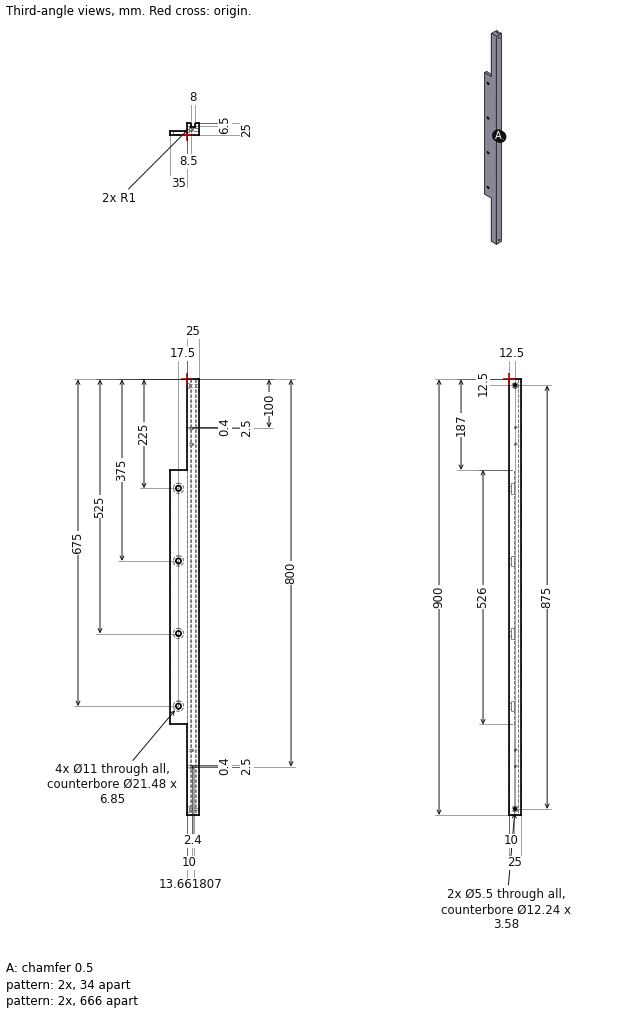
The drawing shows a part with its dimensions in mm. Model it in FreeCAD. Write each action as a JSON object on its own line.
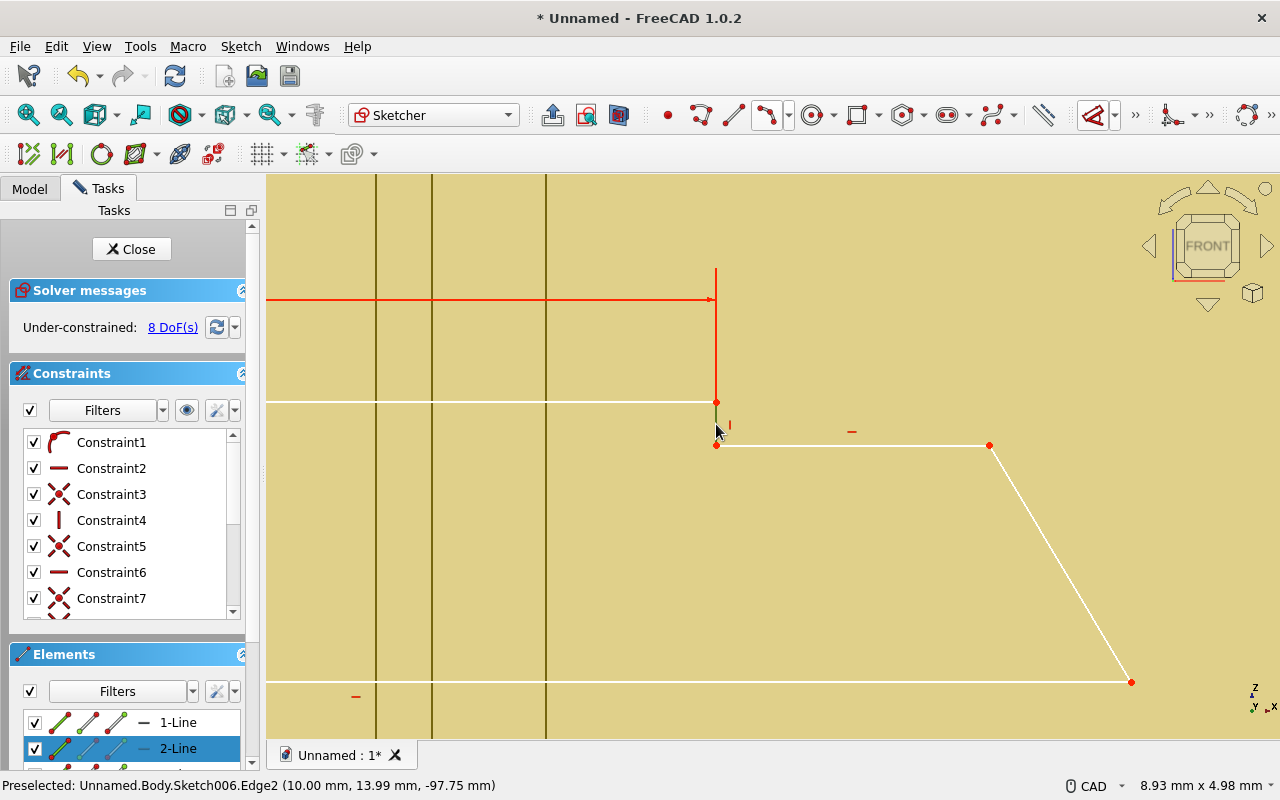
{"action": "left_click", "coordinate": [1114, 116]}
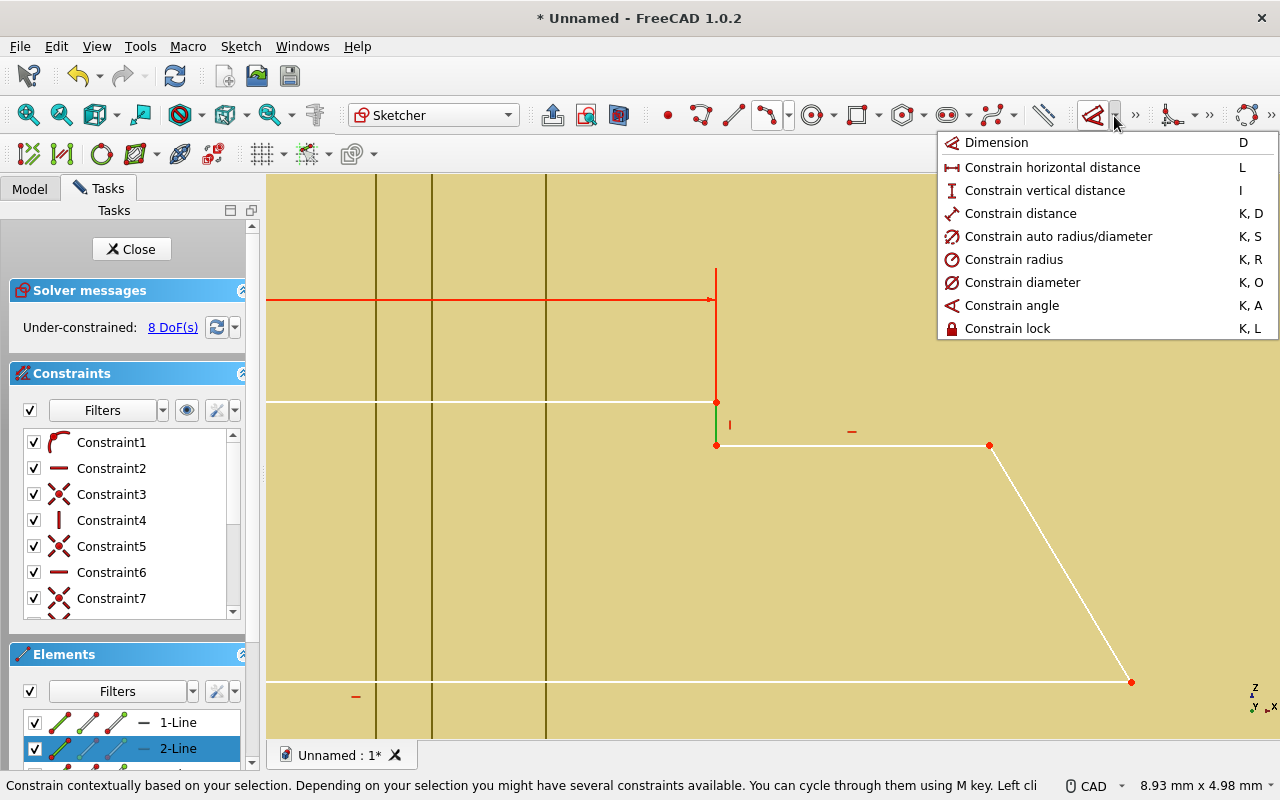
{"action": "left_click", "coordinate": [1108, 190]}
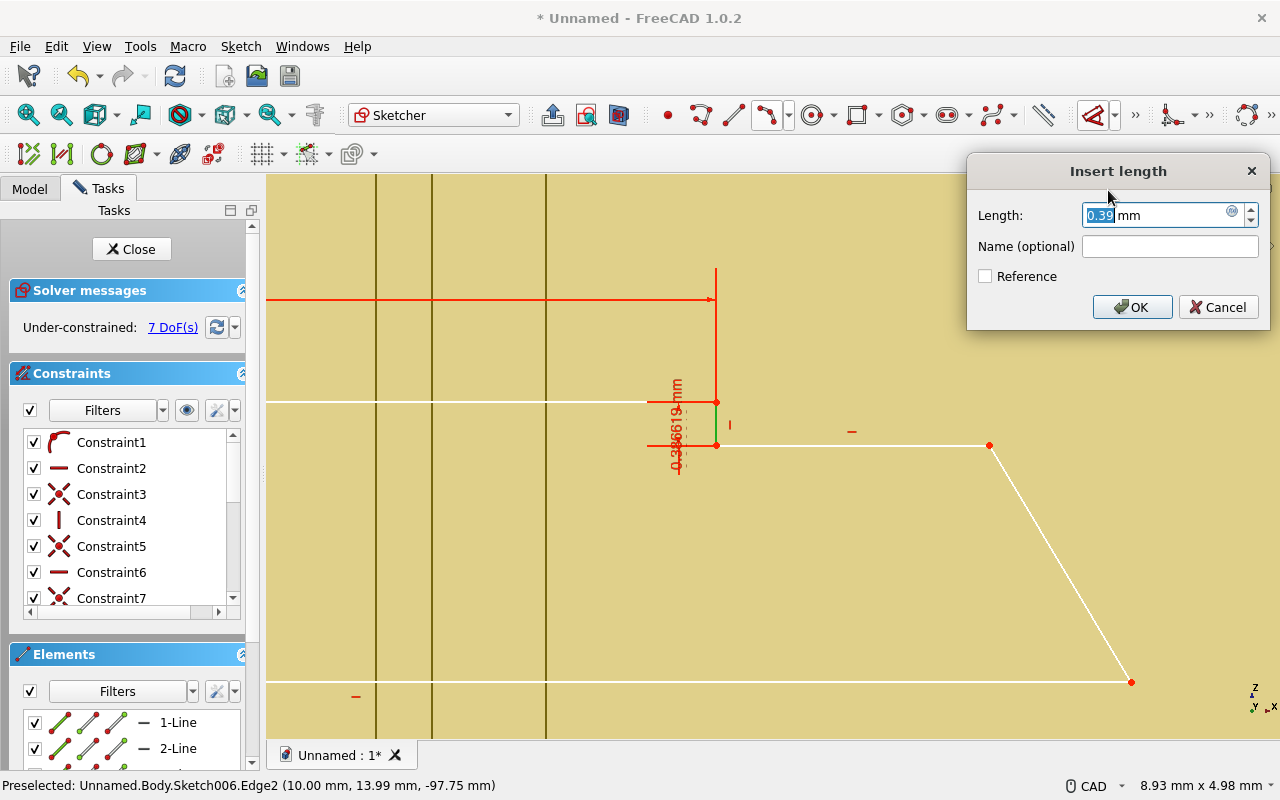
{"action": "type", "text": "0.4"}
{"action": "key", "text": "Return"}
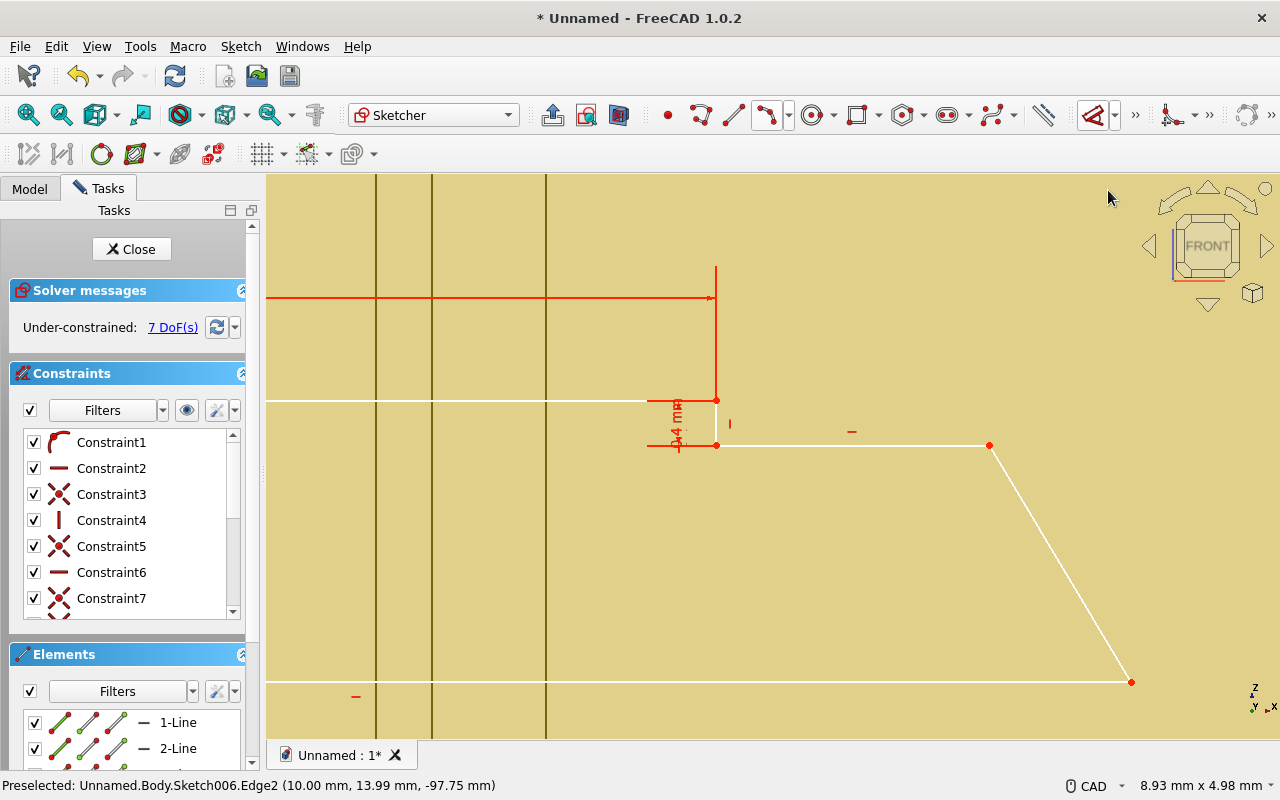
{"action": "scroll", "coordinate": [717, 430], "scroll_direction": "down", "scroll_amount": 7}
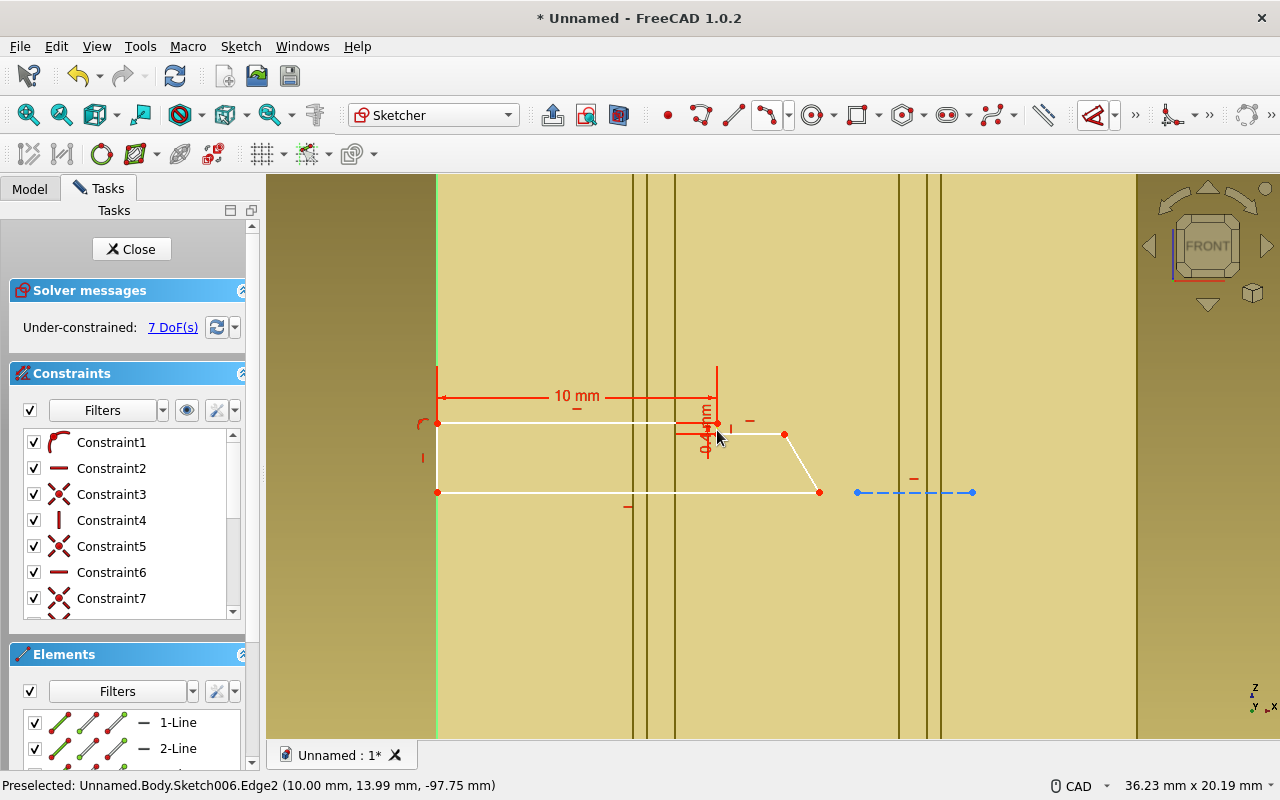
{"action": "left_click", "coordinate": [737, 434]}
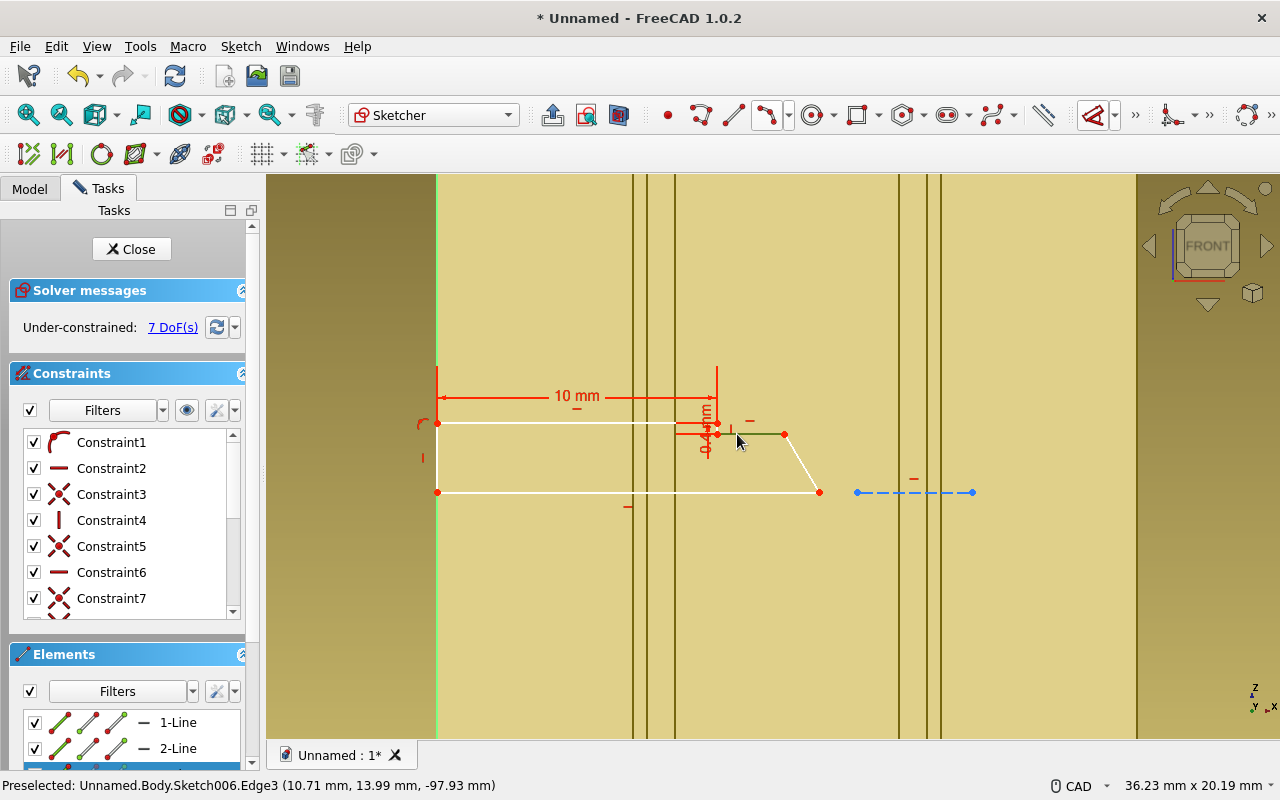
{"action": "left_click", "coordinate": [1114, 116]}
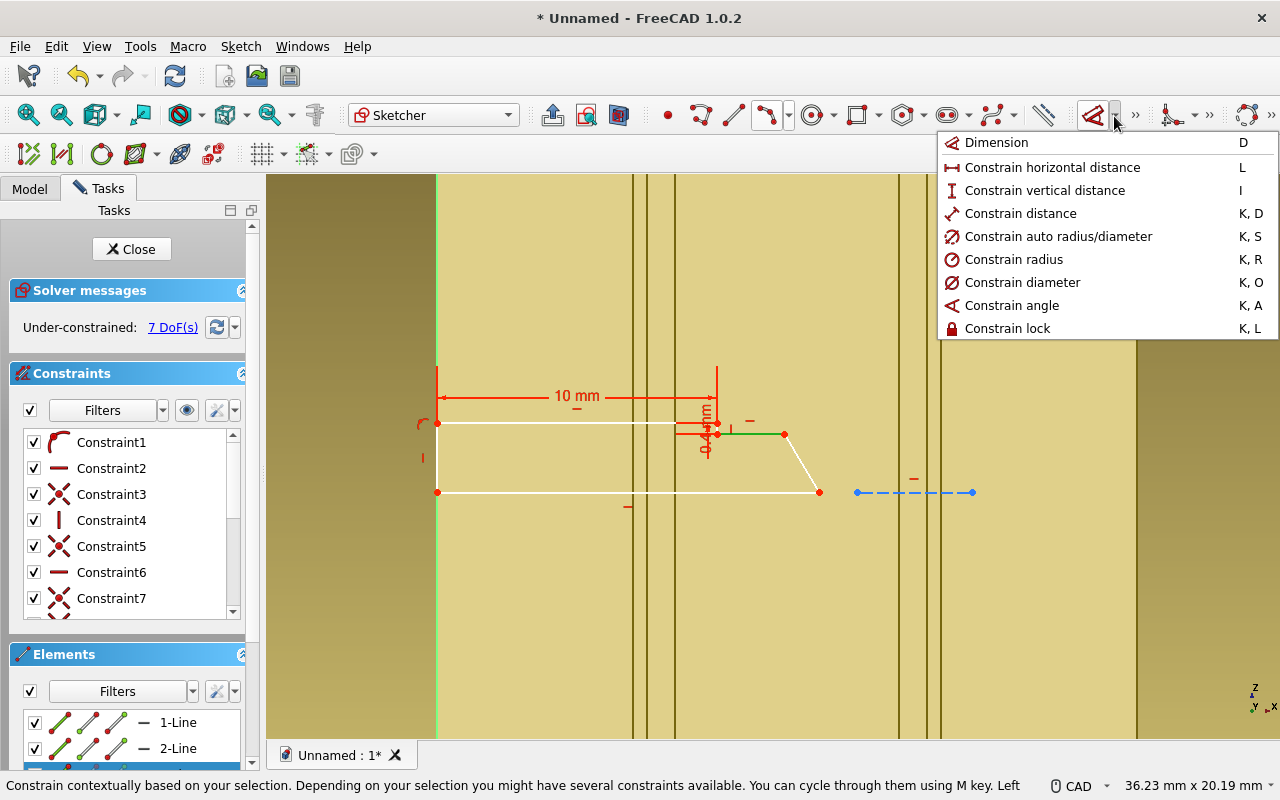
{"action": "left_click", "coordinate": [1108, 168]}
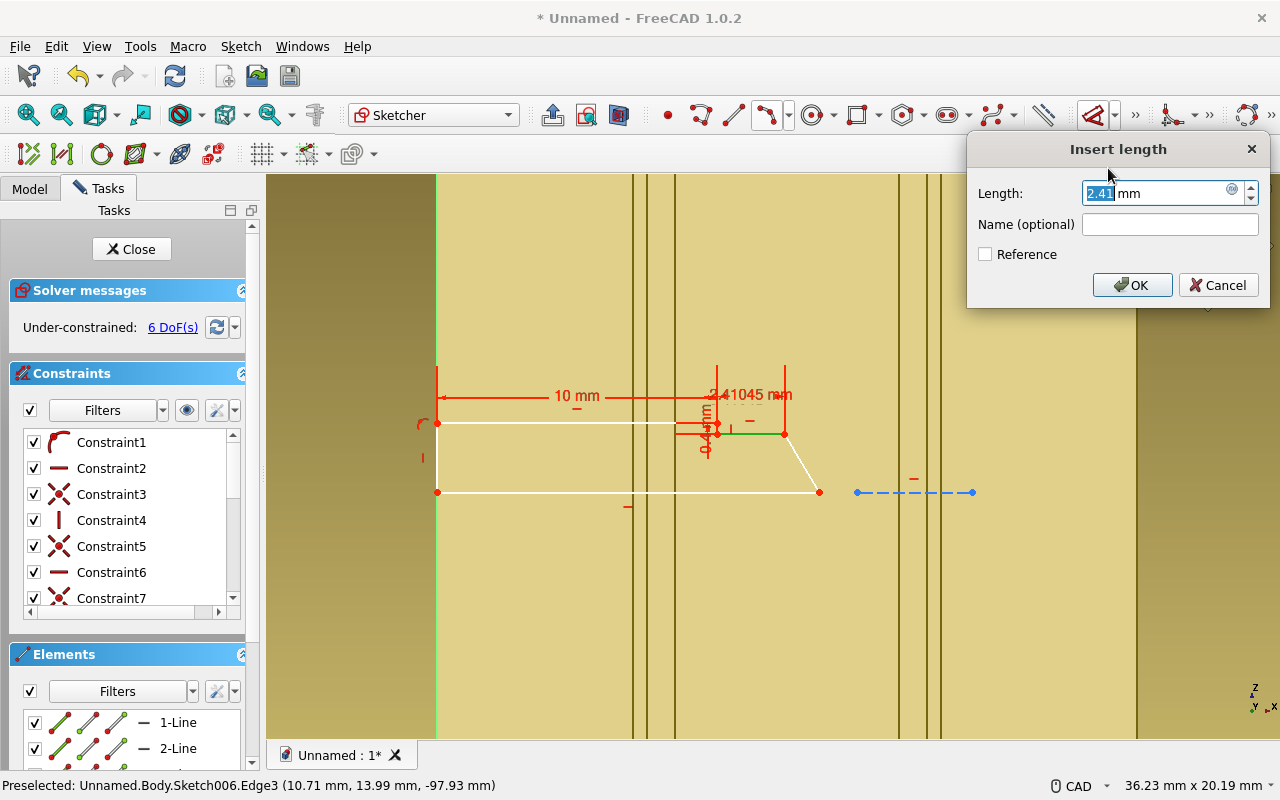
{"action": "type", "text": "2.4"}
{"action": "key", "text": "Return"}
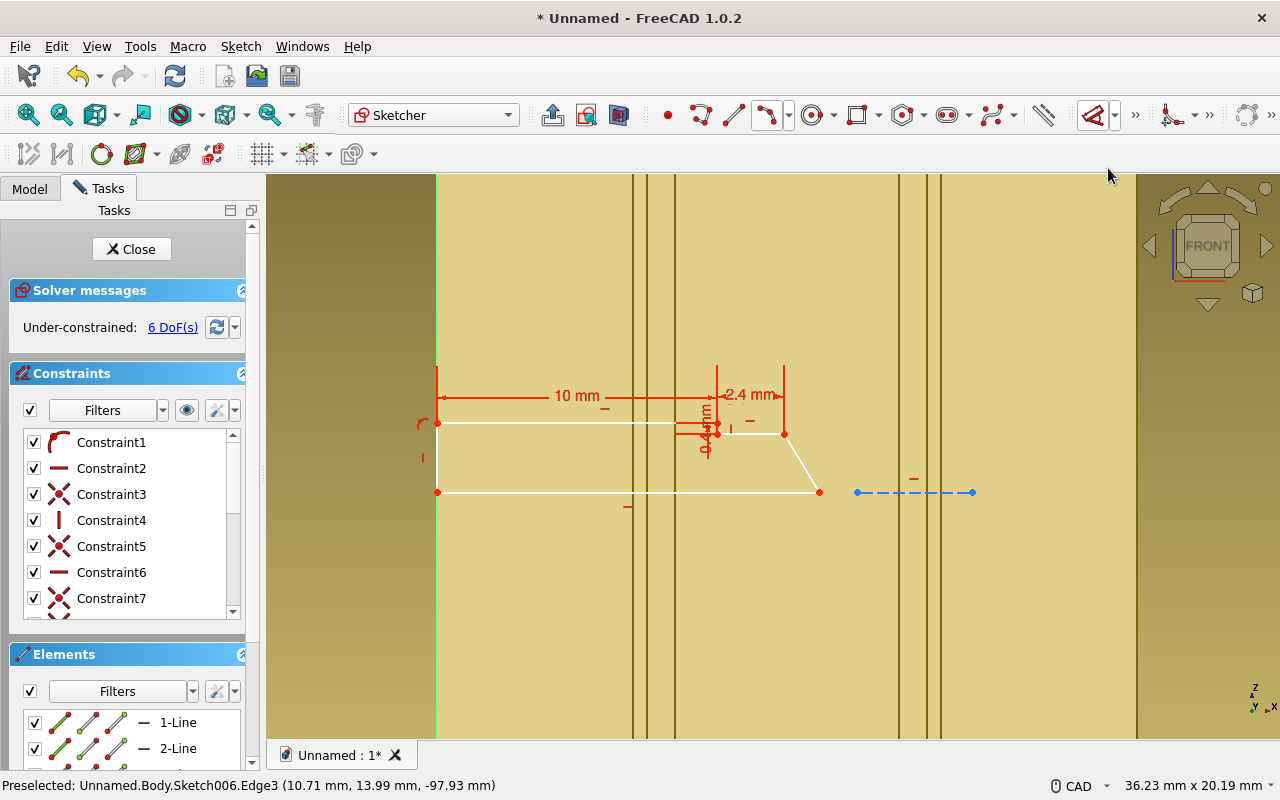
{"action": "left_click", "coordinate": [437, 472]}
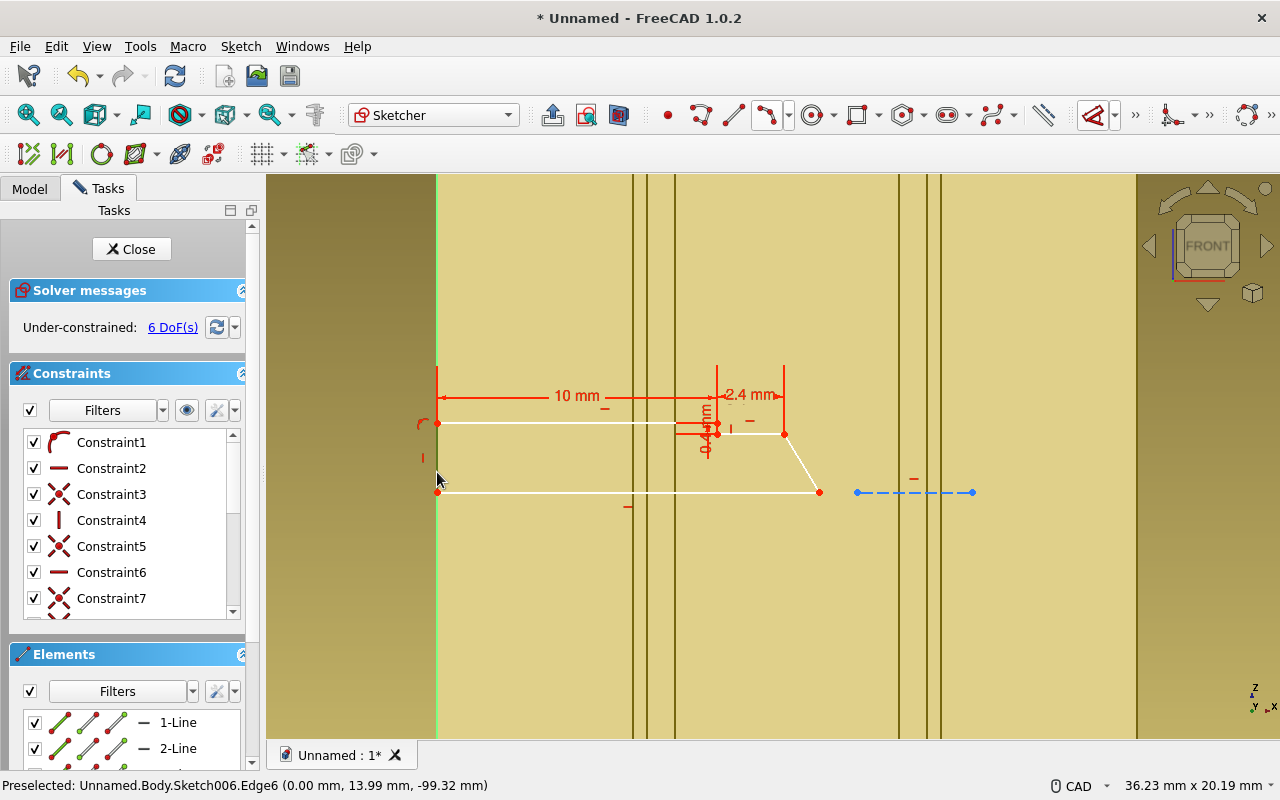
{"action": "key", "text": "i"}